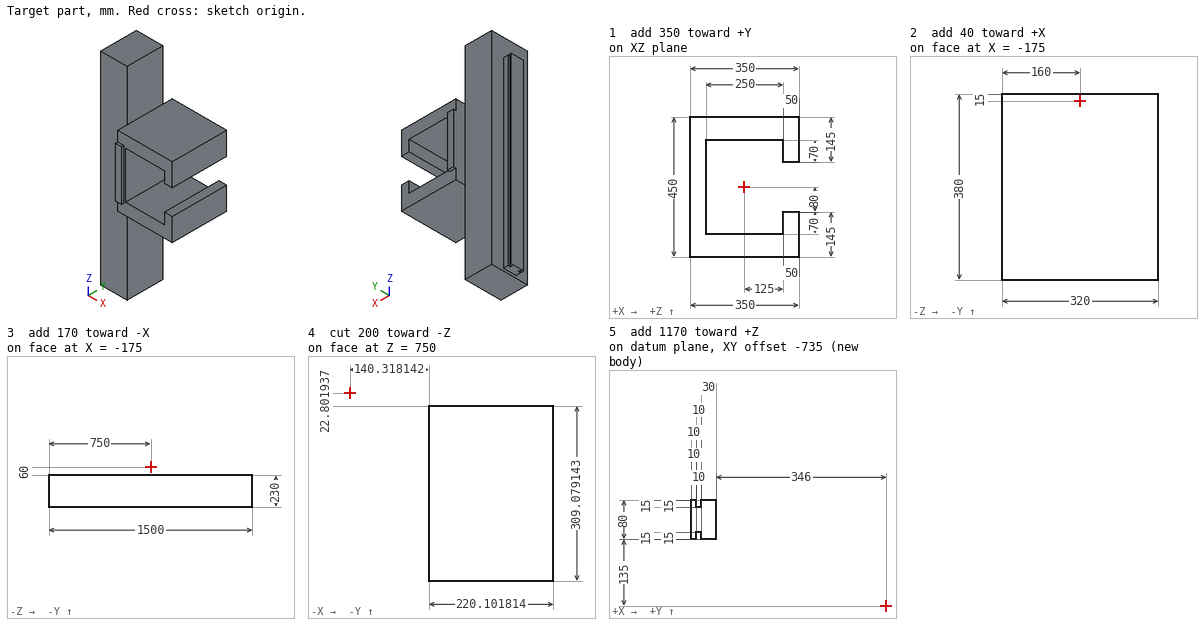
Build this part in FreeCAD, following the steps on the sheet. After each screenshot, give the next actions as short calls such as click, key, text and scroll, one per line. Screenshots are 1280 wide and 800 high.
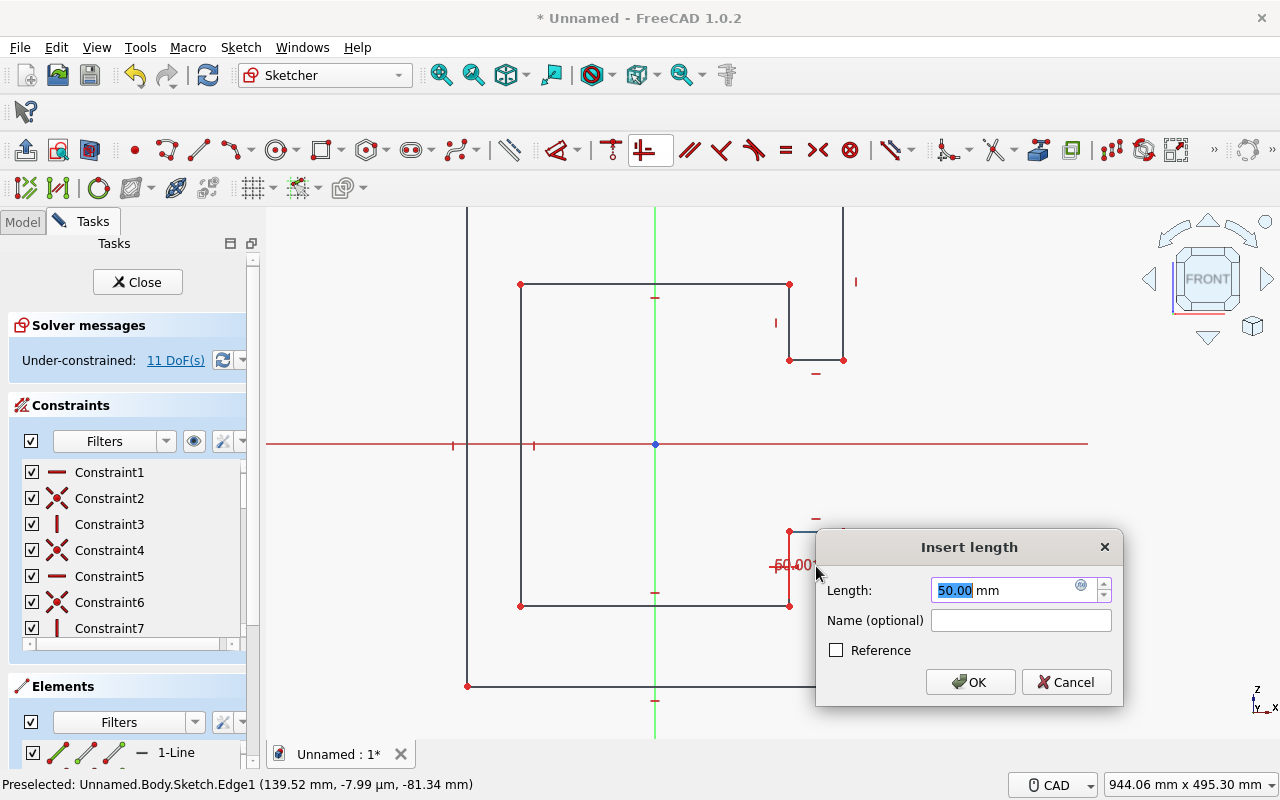
text(50)
key(Return)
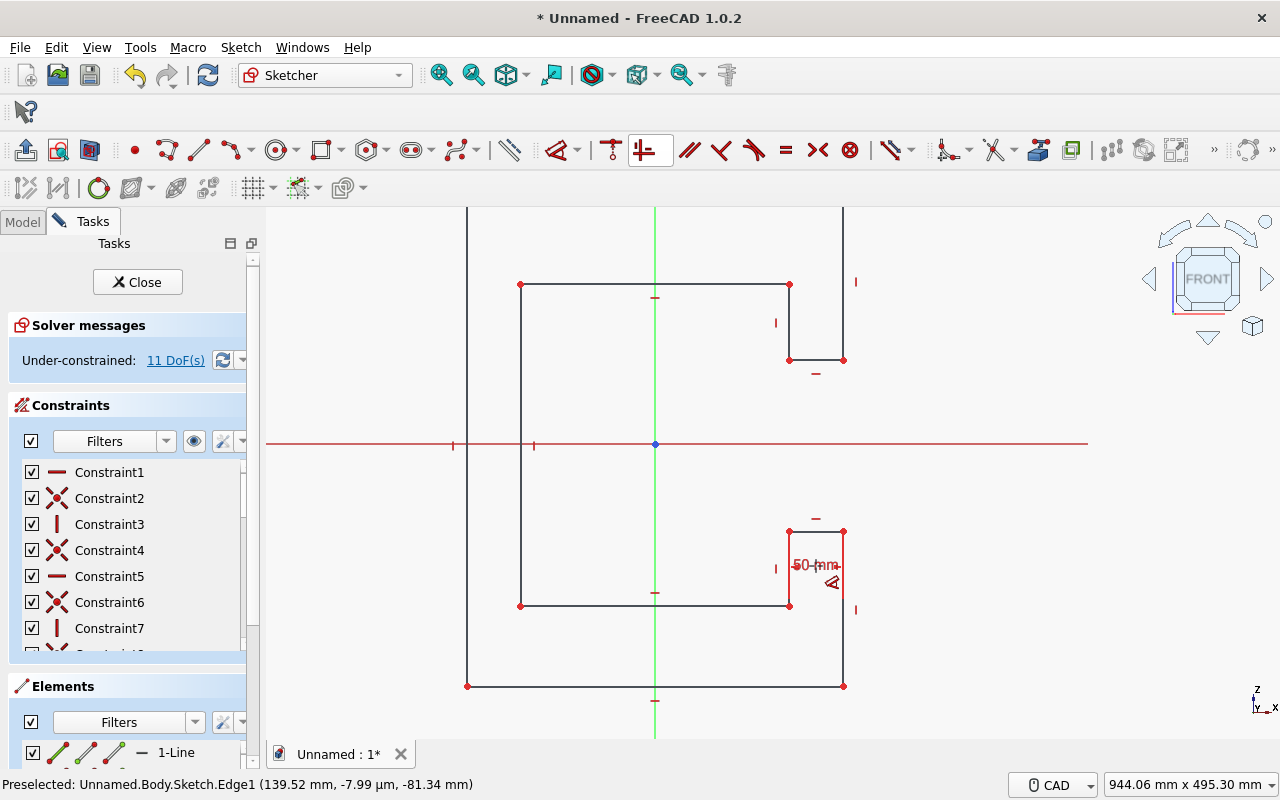
click(827, 360)
click(816, 326)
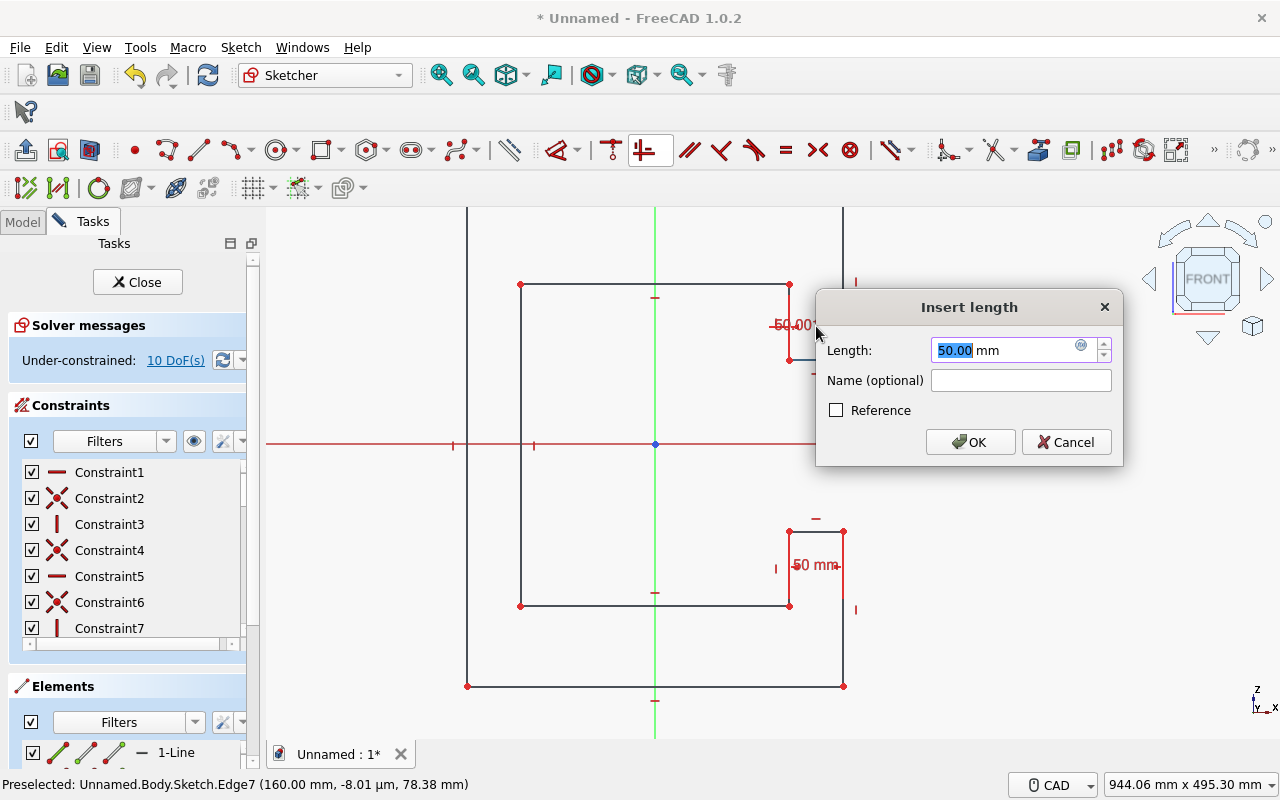
text(50)
key(Return)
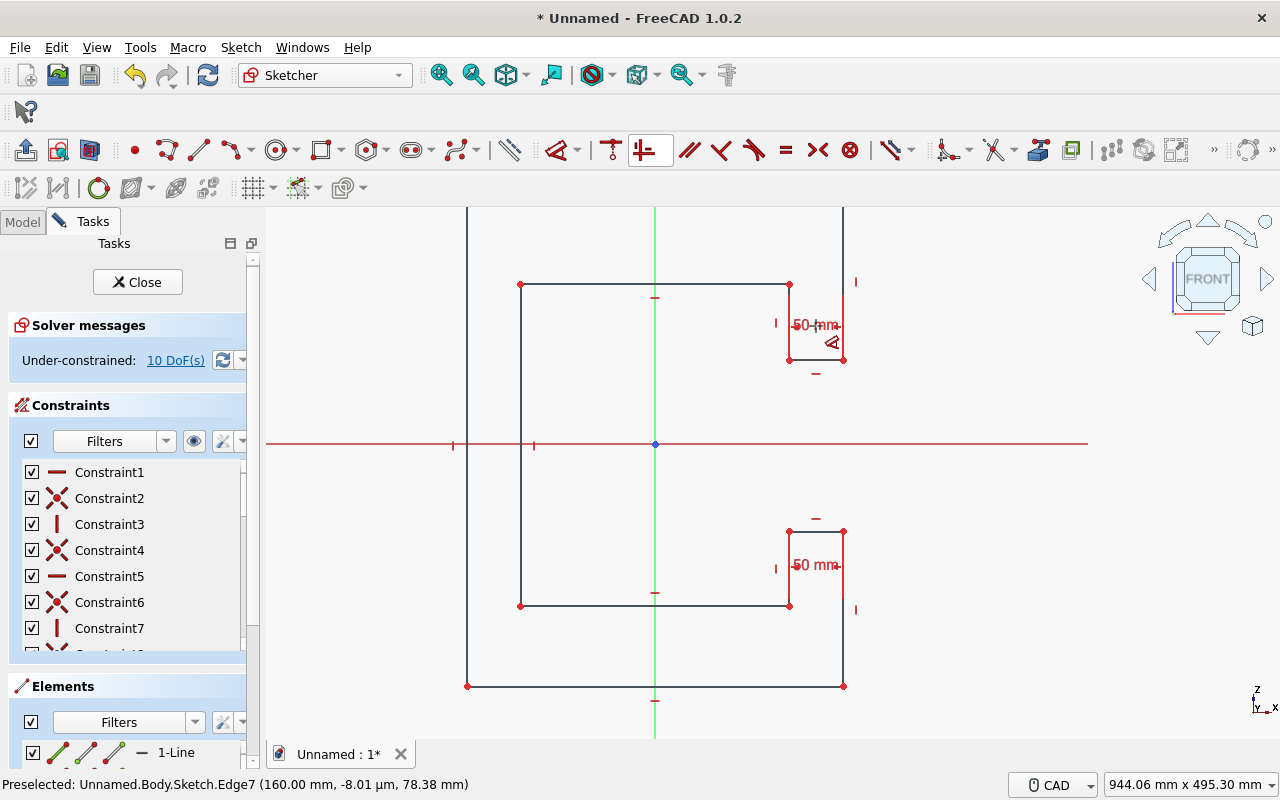
click(789, 337)
click(823, 305)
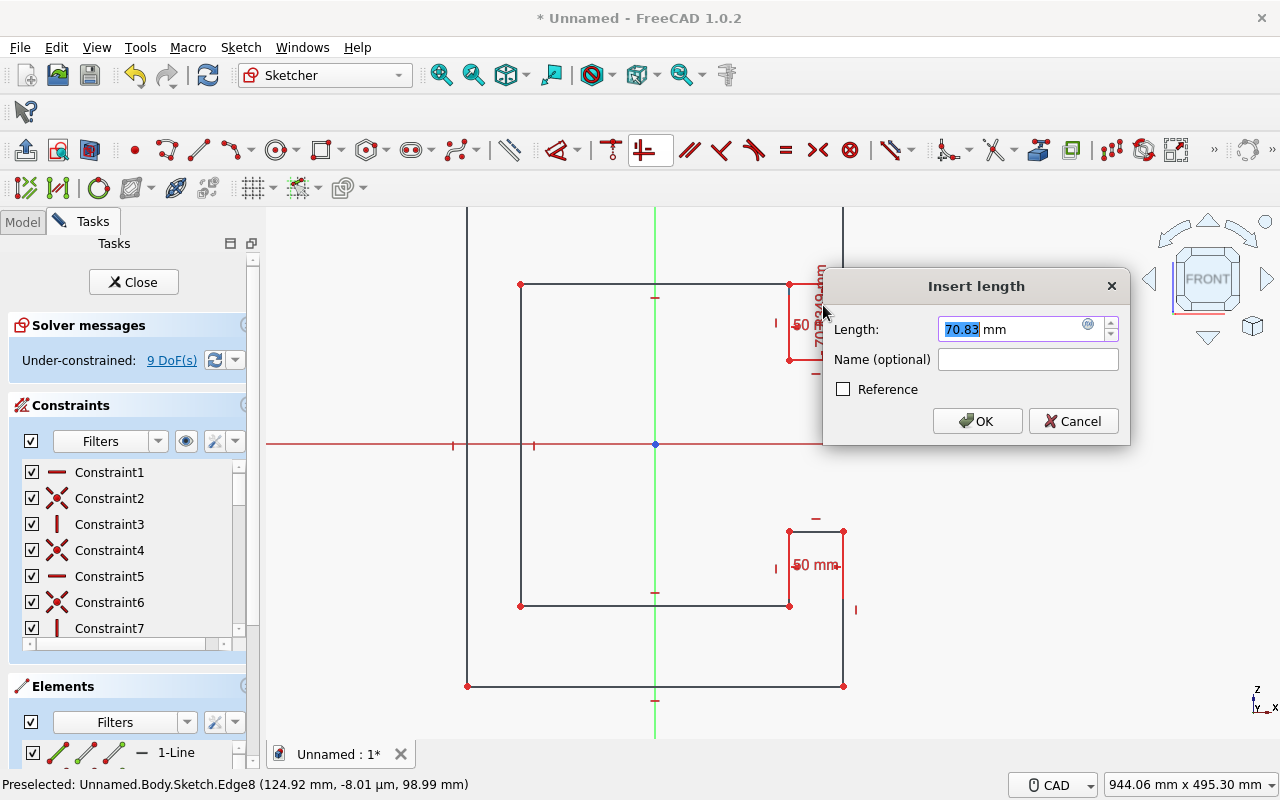
text(70)
key(Return)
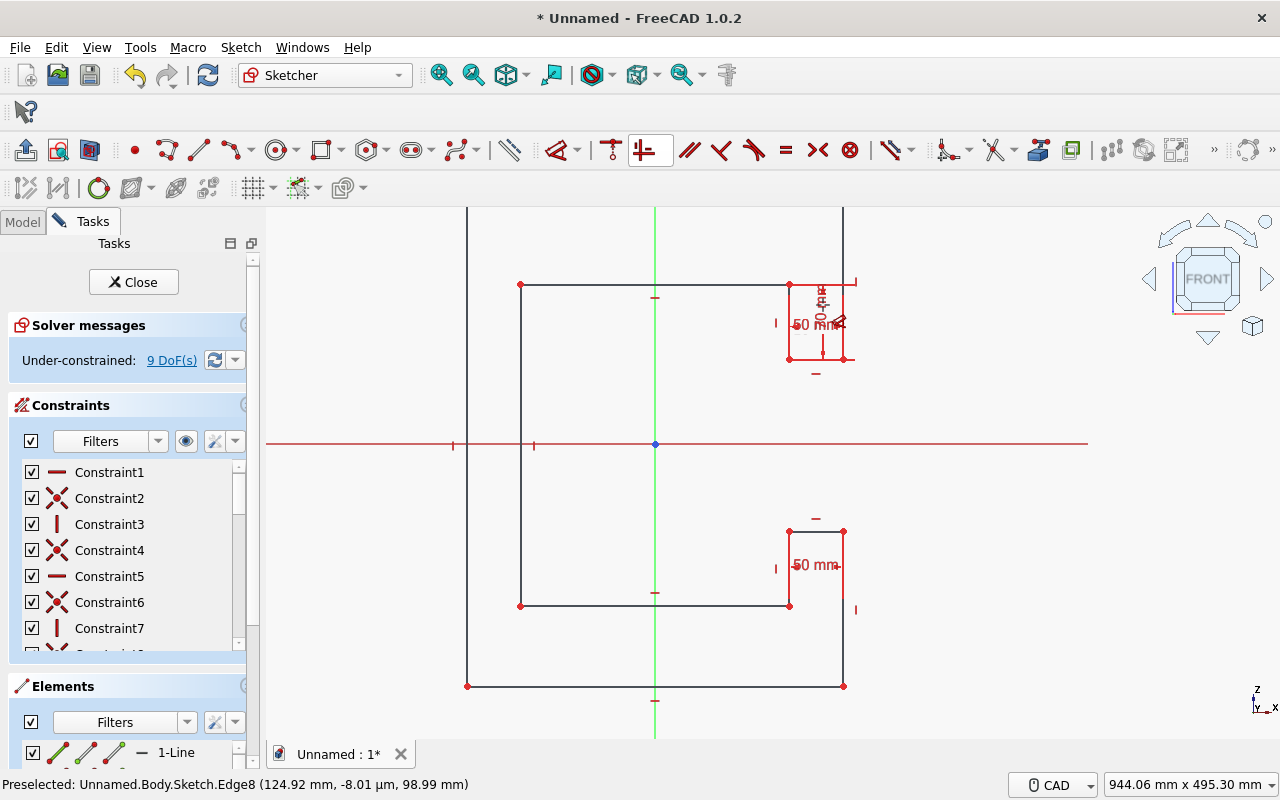
click(789, 584)
click(823, 586)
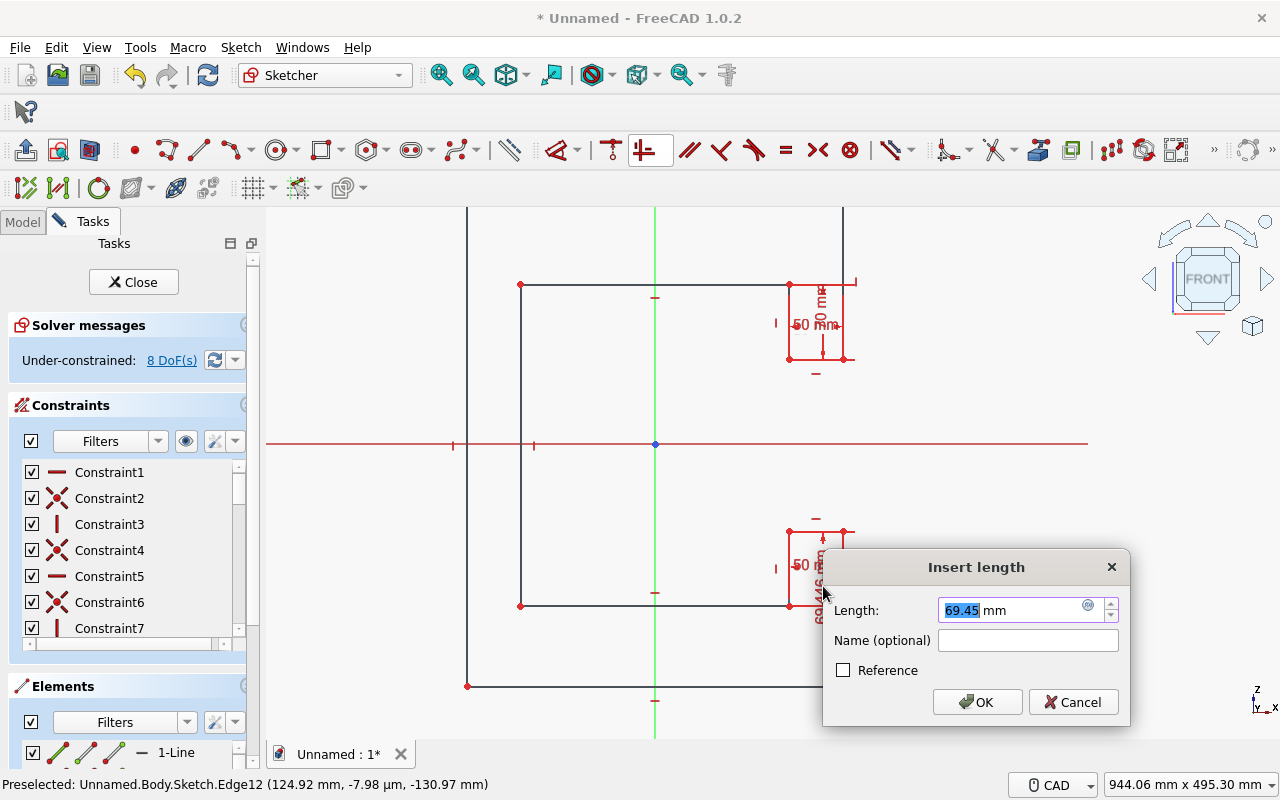
text(70)
key(Return)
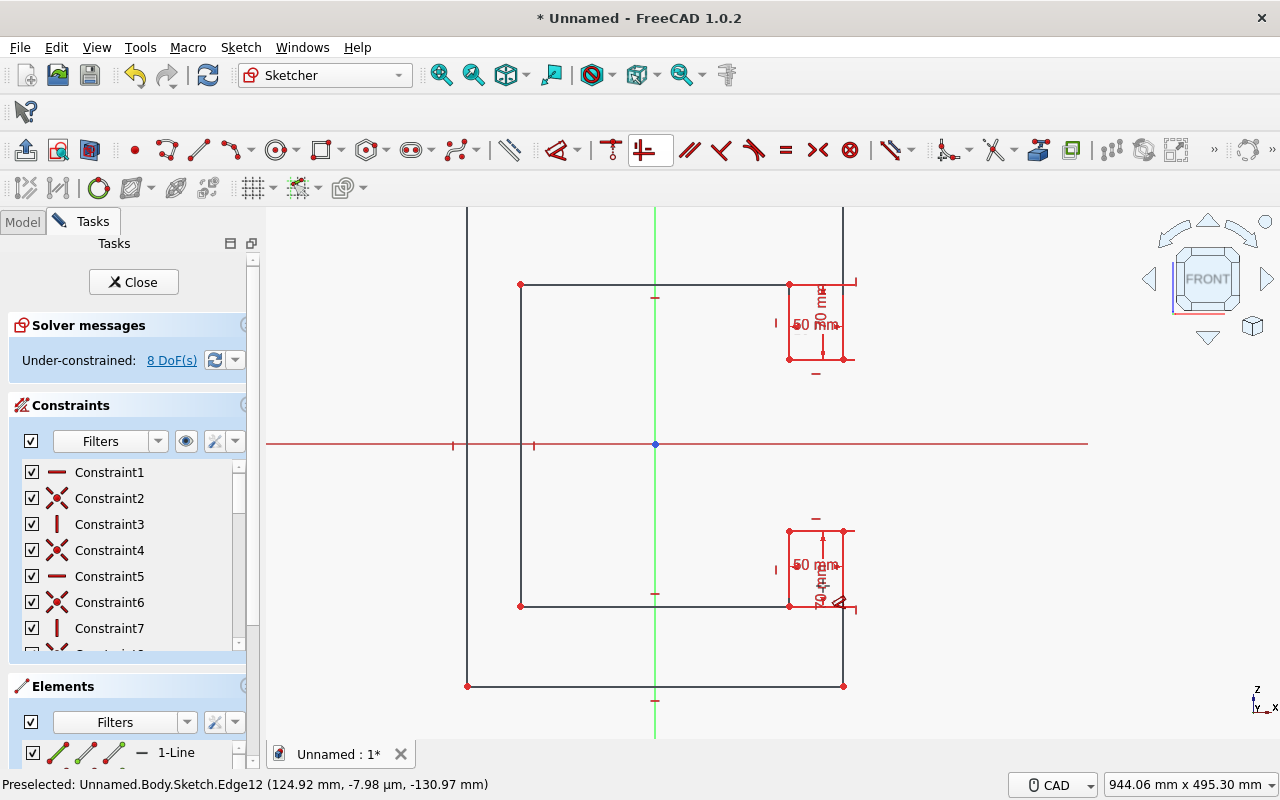
click(843, 578)
click(877, 609)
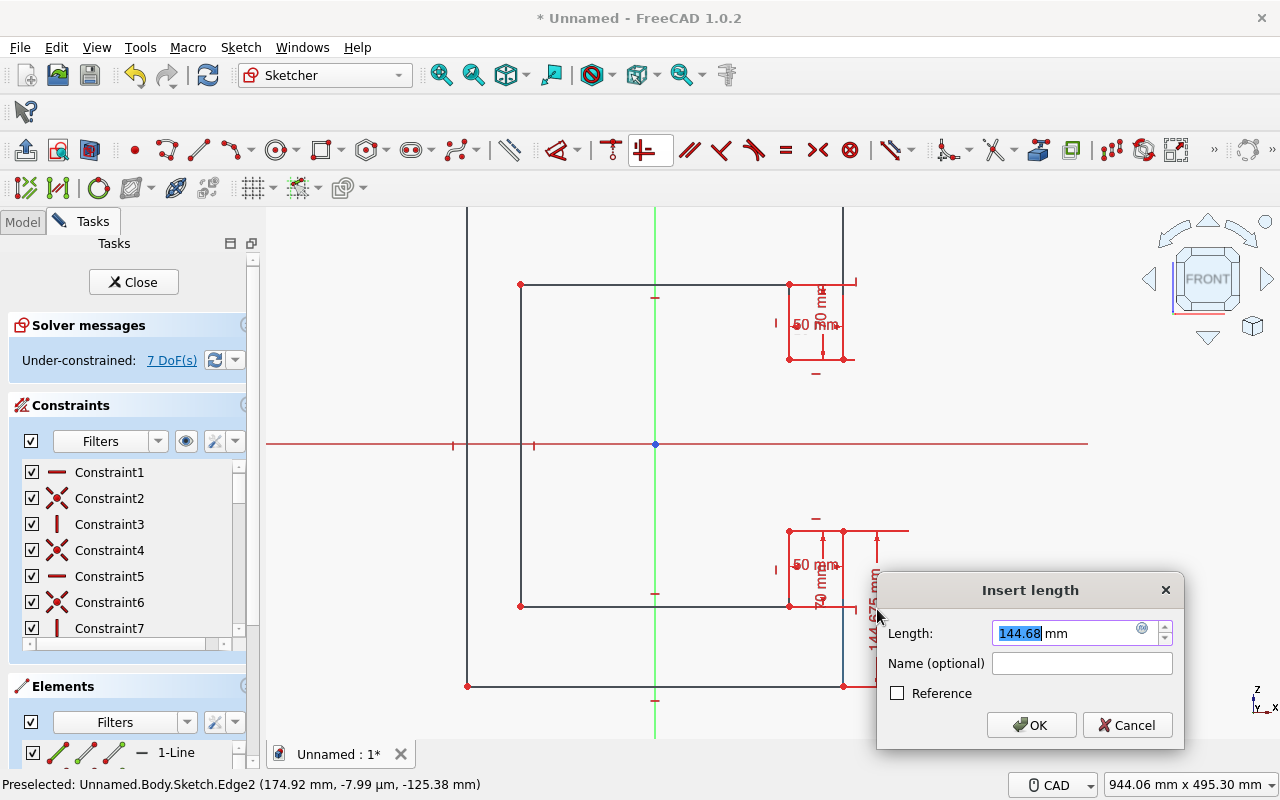
text(145)
key(Return)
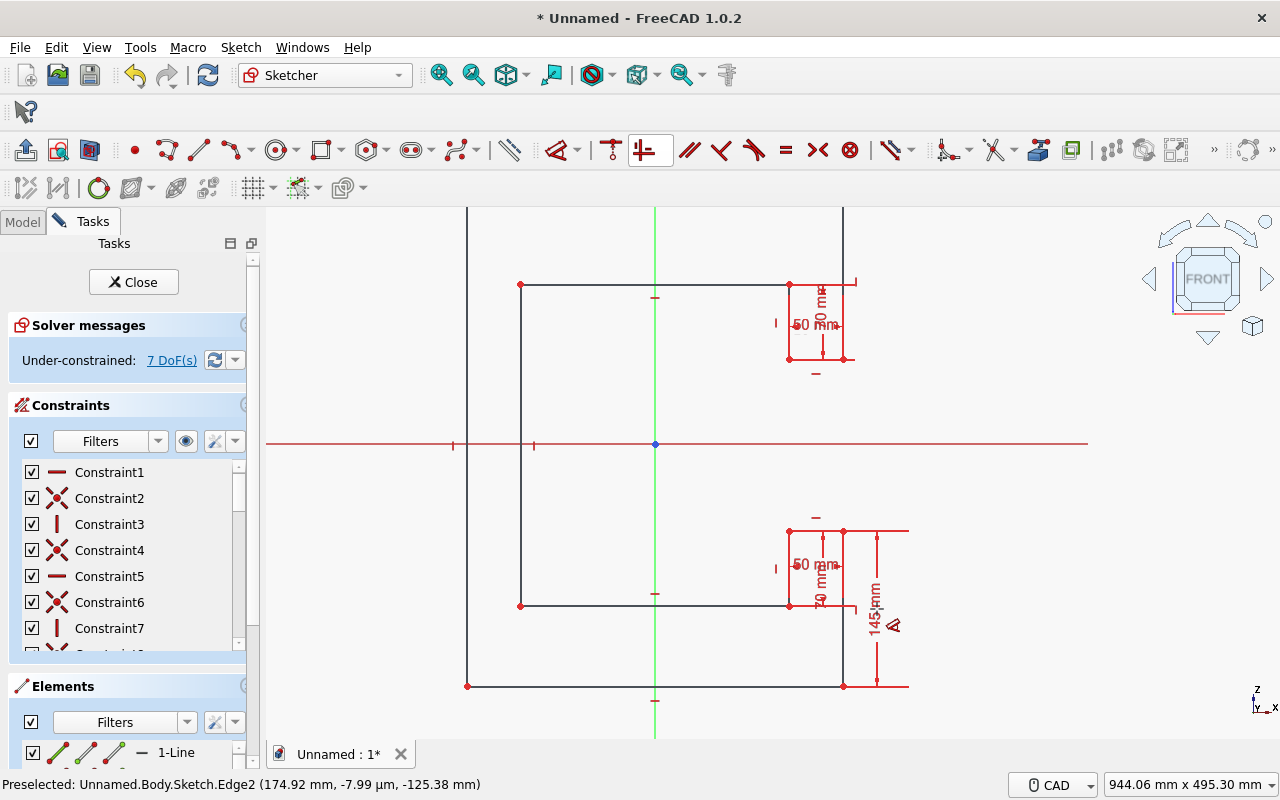
click(730, 687)
click(569, 653)